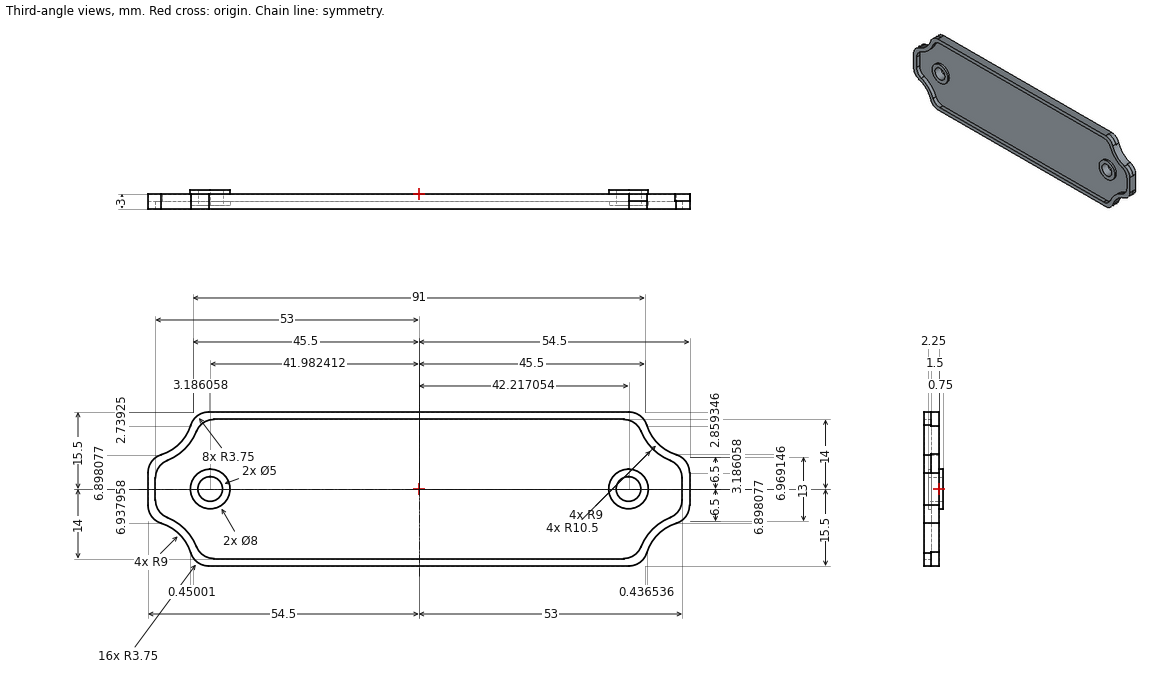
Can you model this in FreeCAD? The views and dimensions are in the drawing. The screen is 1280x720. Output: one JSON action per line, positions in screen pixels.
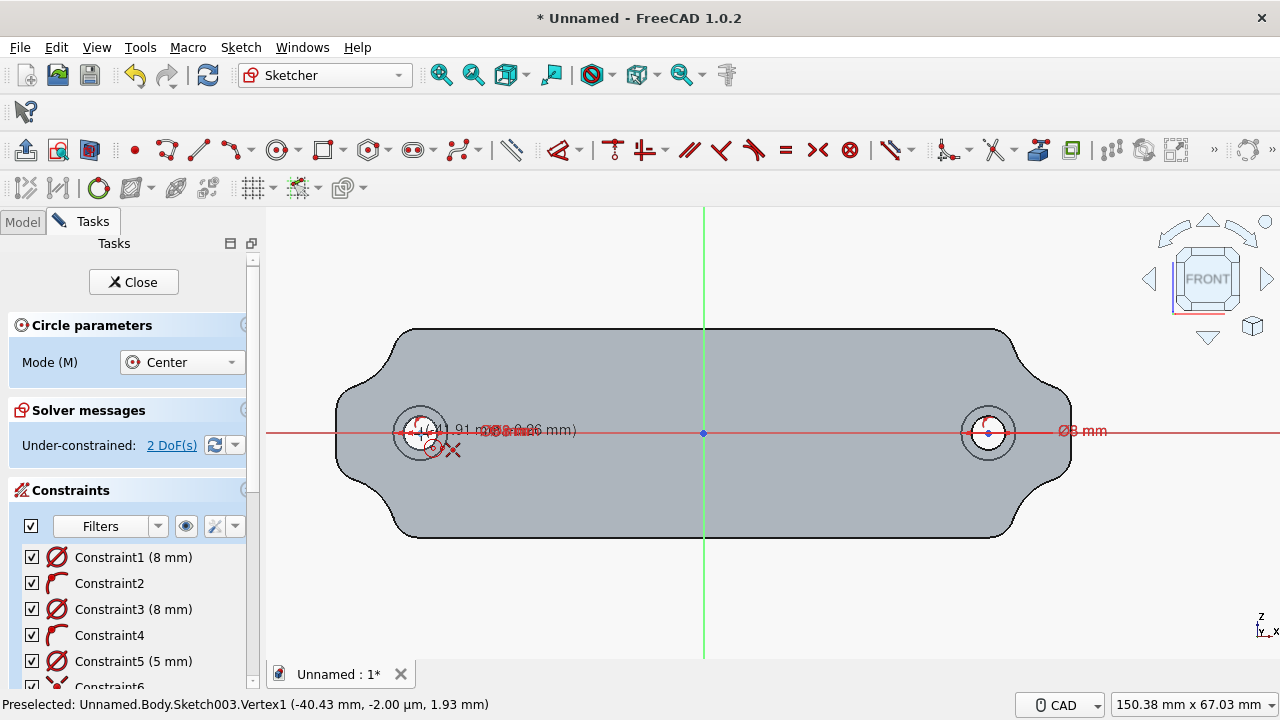
{"action": "scroll", "coordinate": [988, 433], "scroll_direction": "up", "scroll_amount": 2}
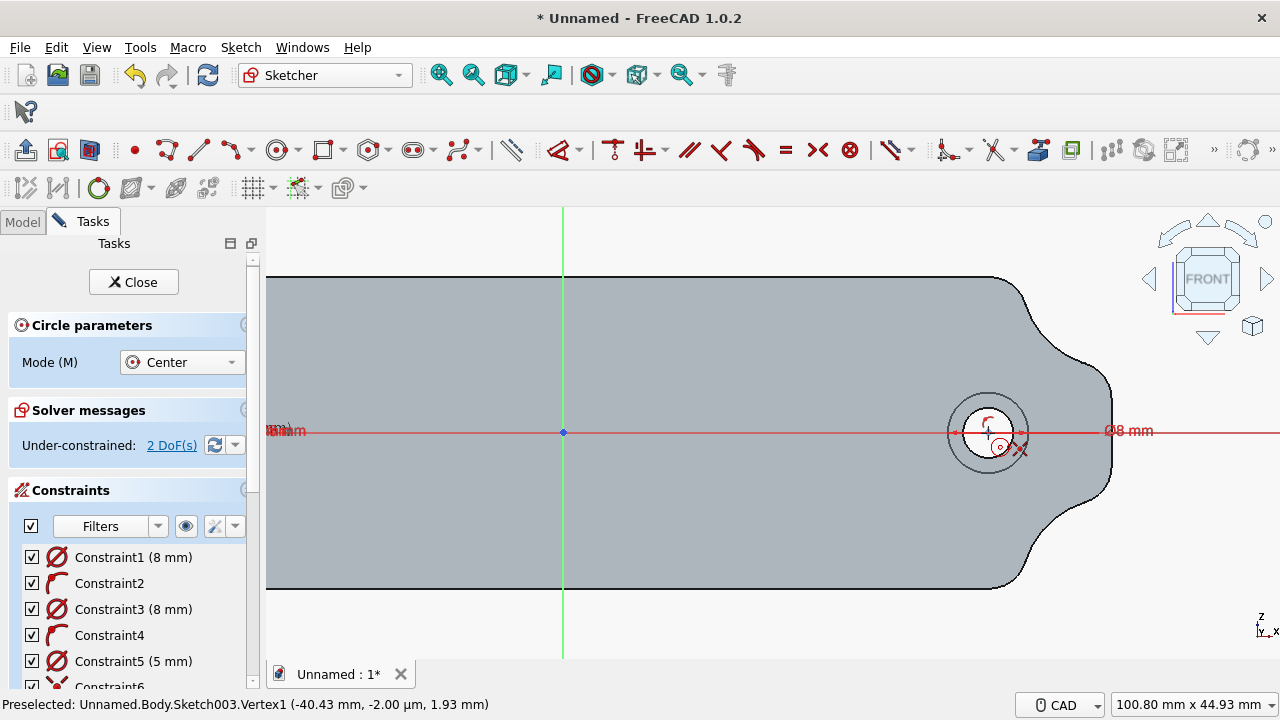
{"action": "left_click", "coordinate": [988, 433]}
{"action": "mouse_move", "coordinate": [1006, 415]}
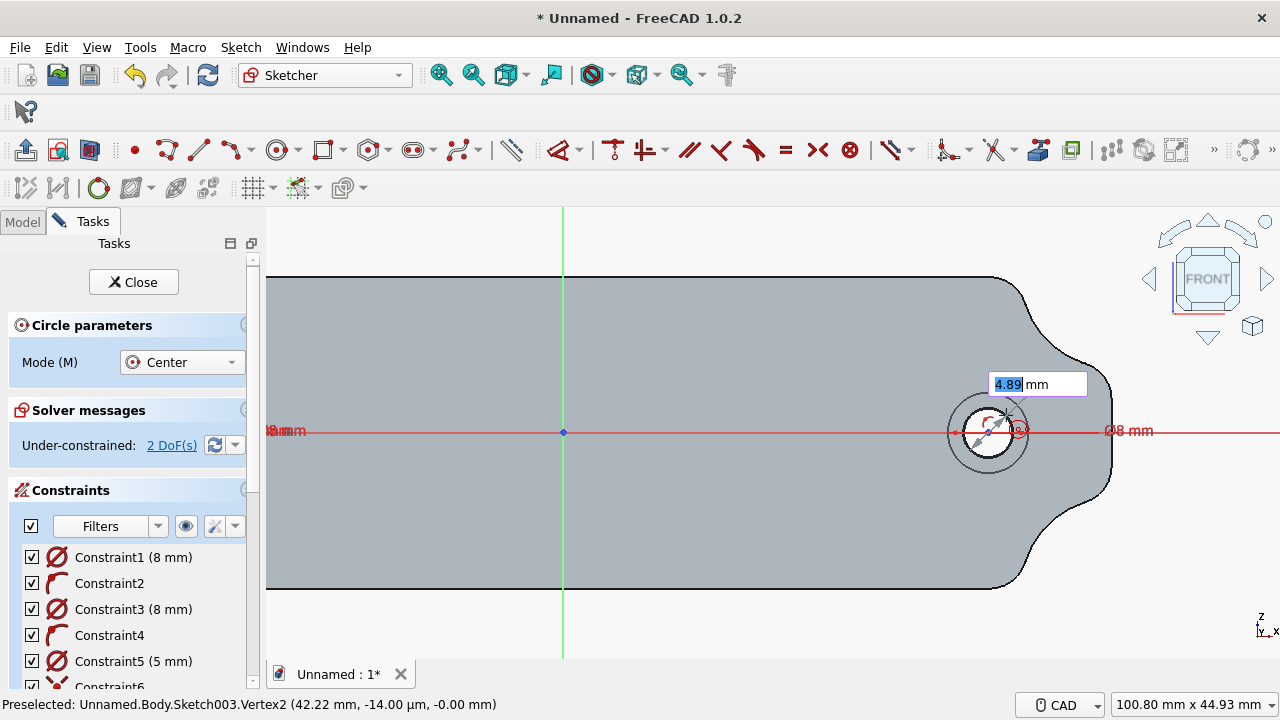
{"action": "type", "text": "5"}
{"action": "key", "text": "Return"}
{"action": "key", "text": "Escape"}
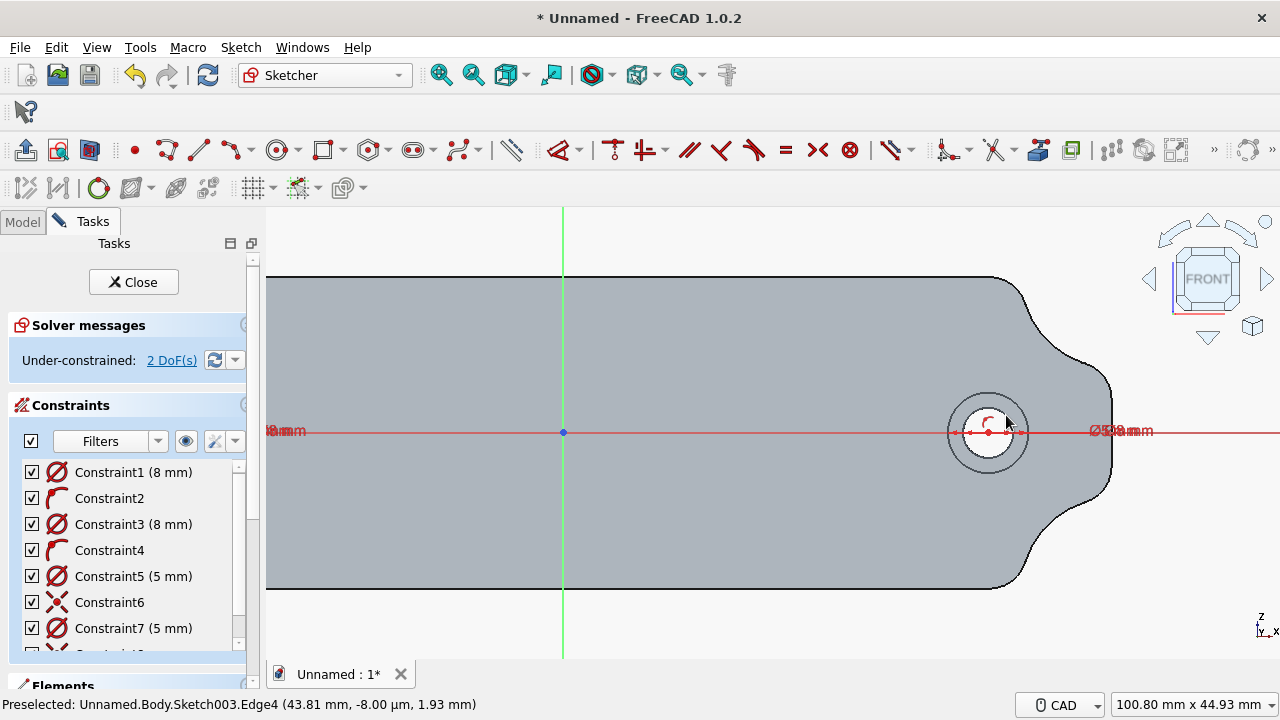
{"action": "left_click", "coordinate": [558, 150]}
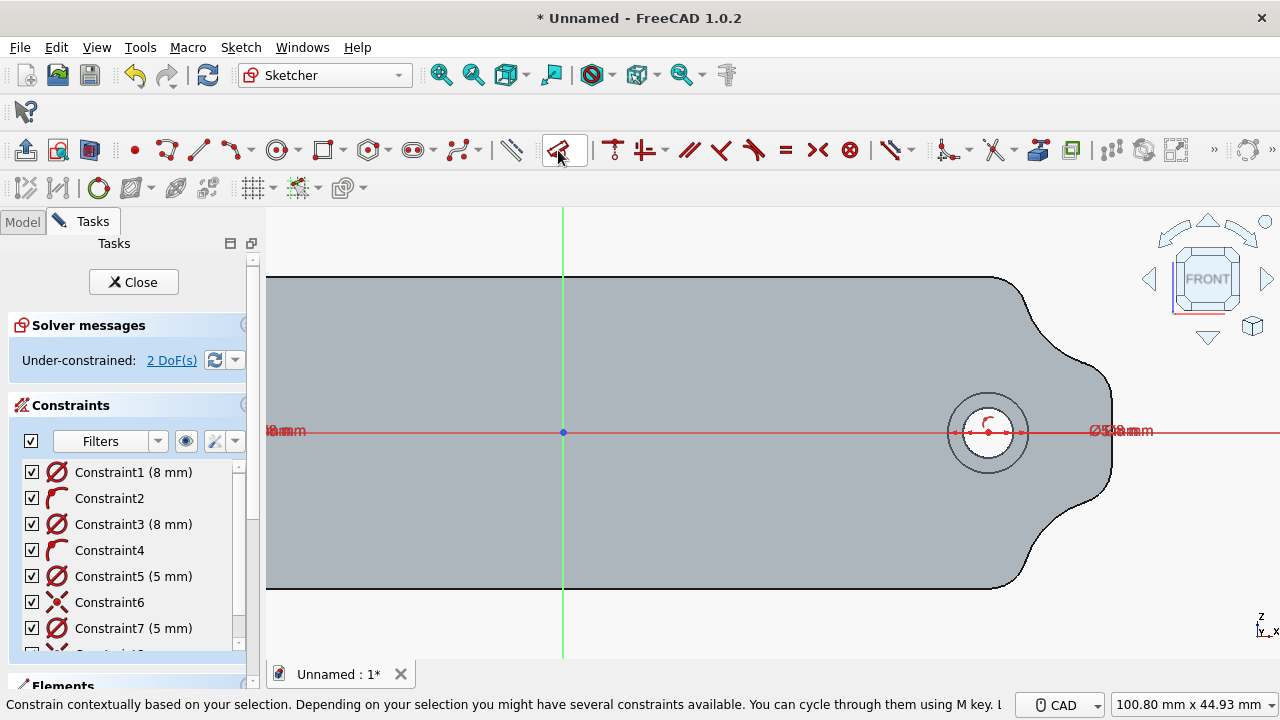
{"action": "scroll", "coordinate": [989, 433], "scroll_direction": "down", "scroll_amount": 2}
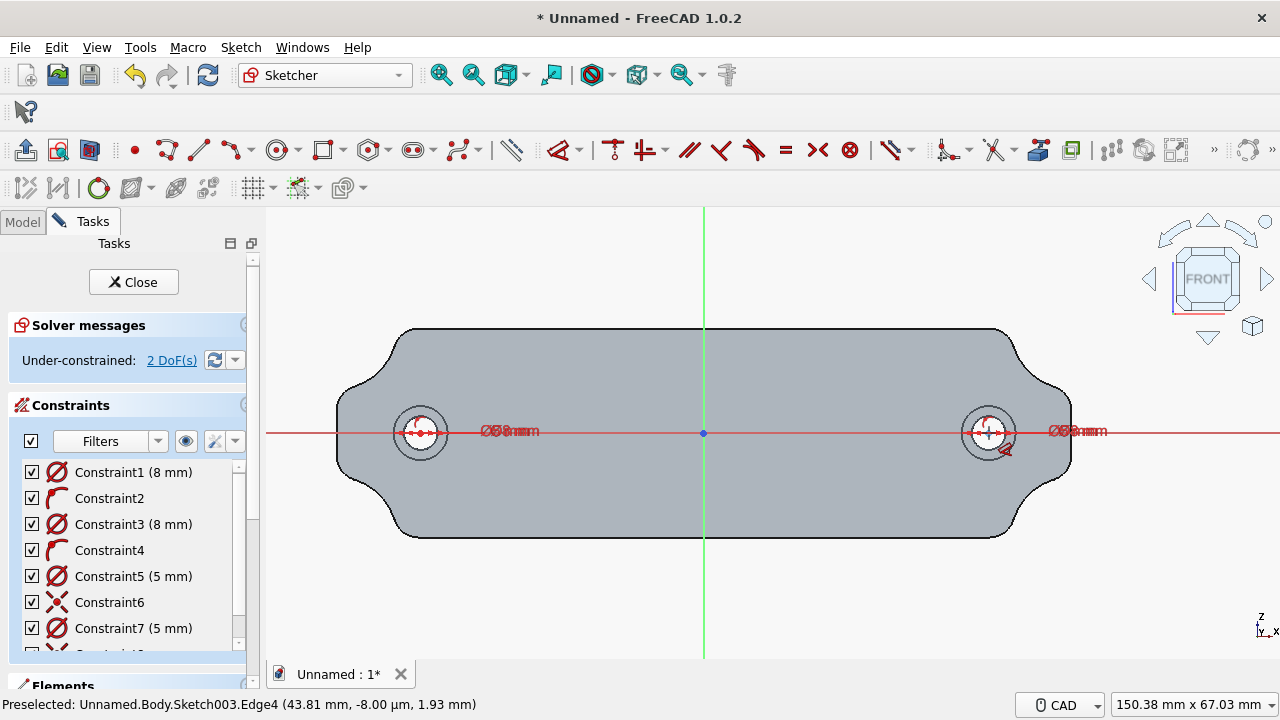
{"action": "left_click", "coordinate": [421, 433]}
{"action": "left_click", "coordinate": [562, 467]}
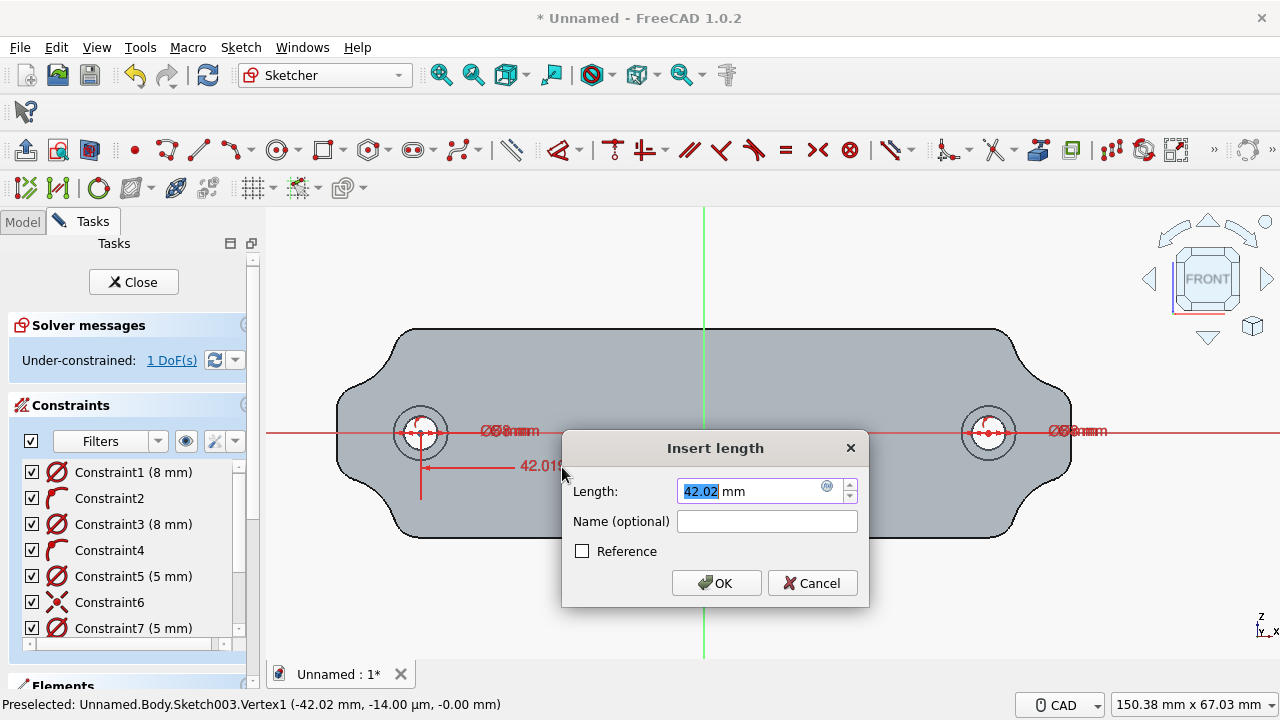
{"action": "type", "text": "41.982412"}
{"action": "key", "text": "Return"}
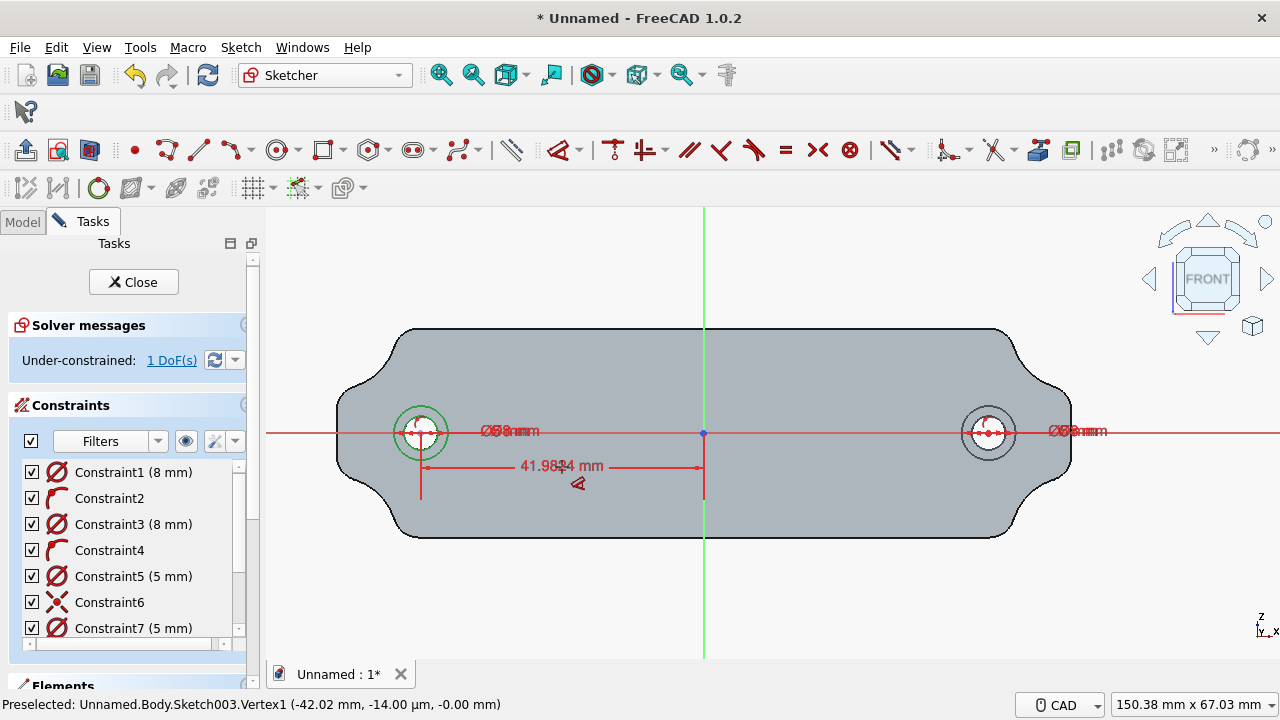
{"action": "left_click", "coordinate": [989, 433]}
{"action": "left_click", "coordinate": [846, 467]}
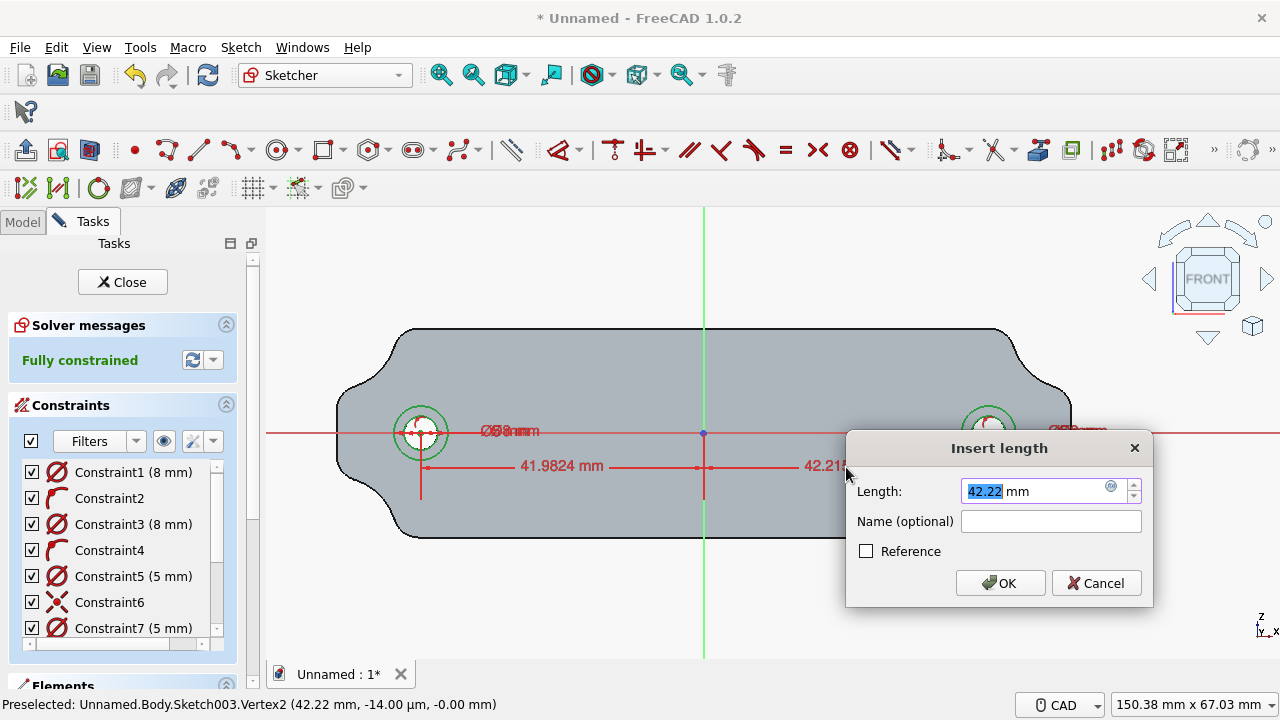
{"action": "type", "text": "42.217054"}
{"action": "key", "text": "Return"}
{"action": "key", "text": "Escape"}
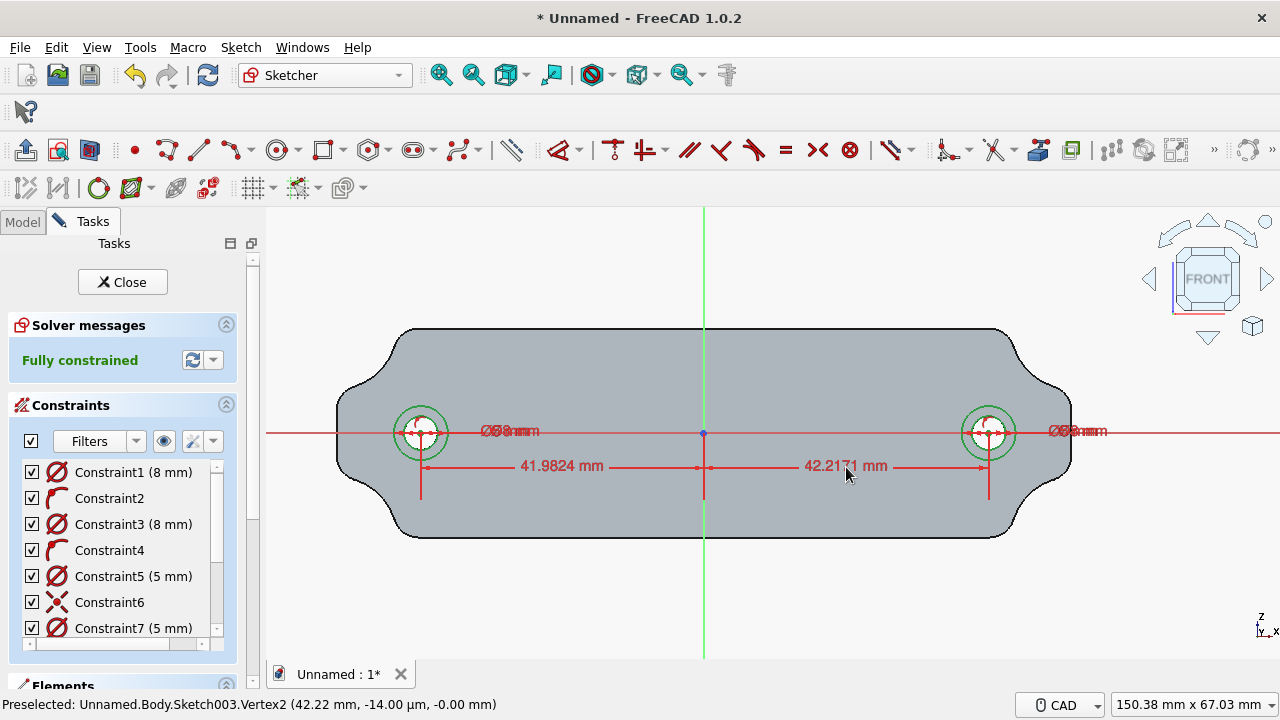
{"action": "left_click", "coordinate": [123, 282]}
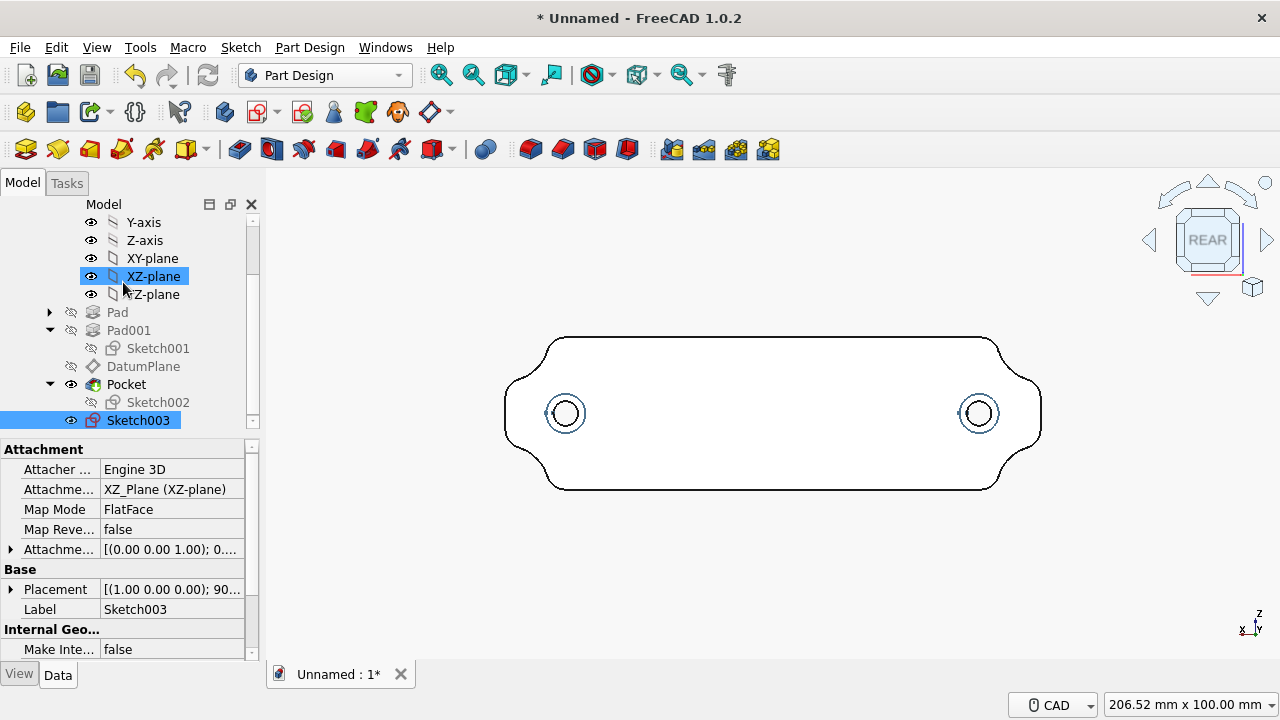
{"action": "left_click", "coordinate": [26, 150]}